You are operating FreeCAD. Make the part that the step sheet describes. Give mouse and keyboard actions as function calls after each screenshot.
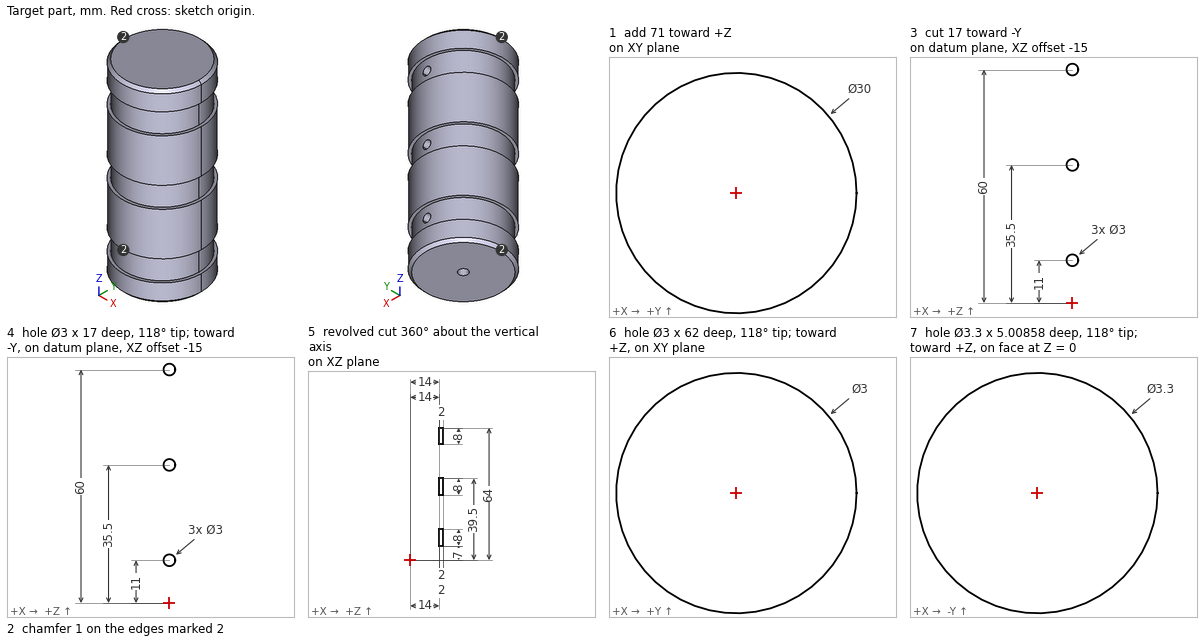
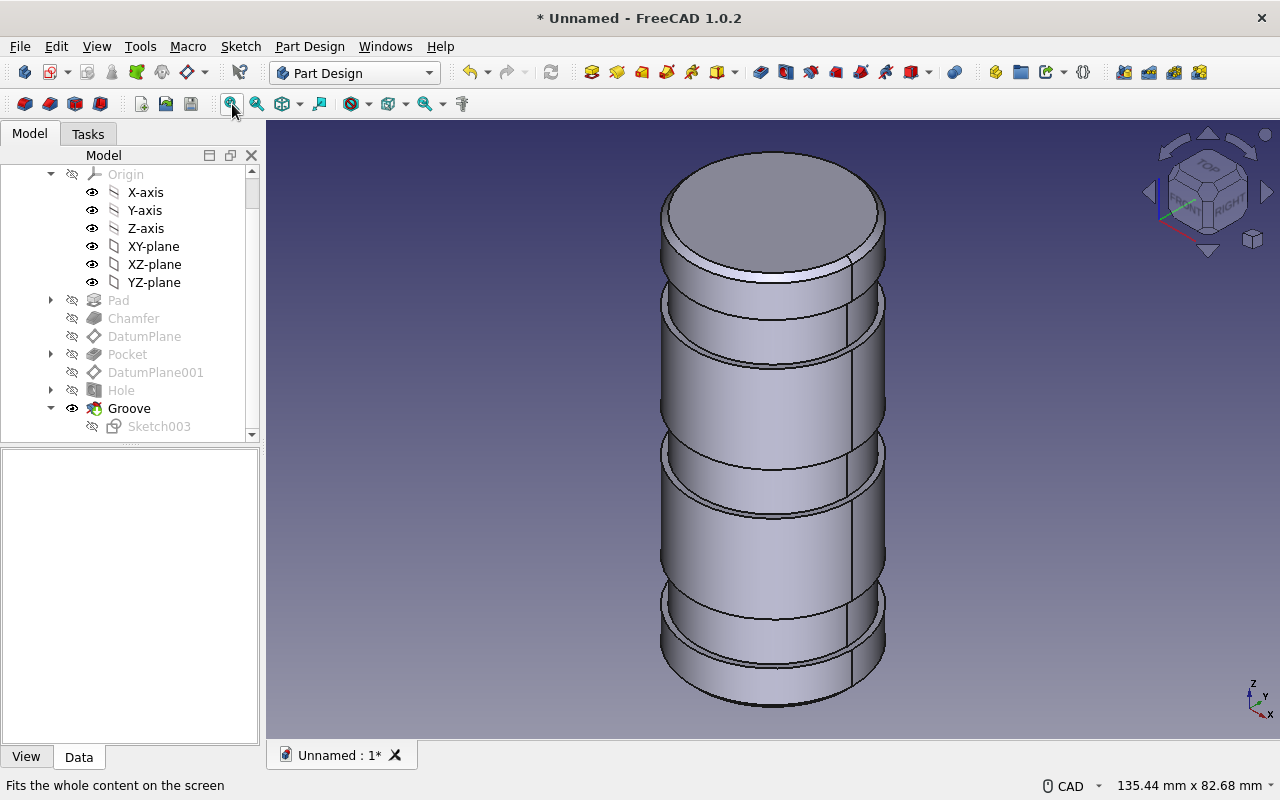
click(50, 72)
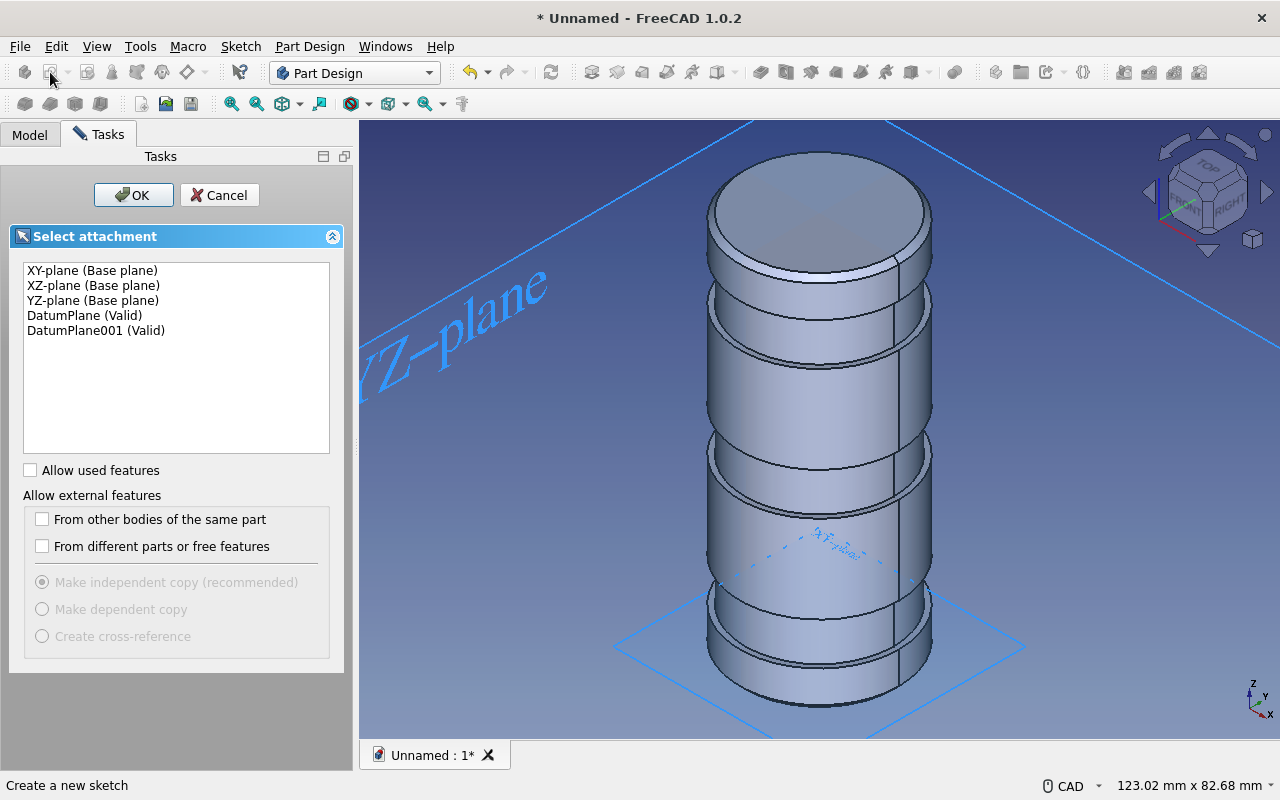
click(84, 270)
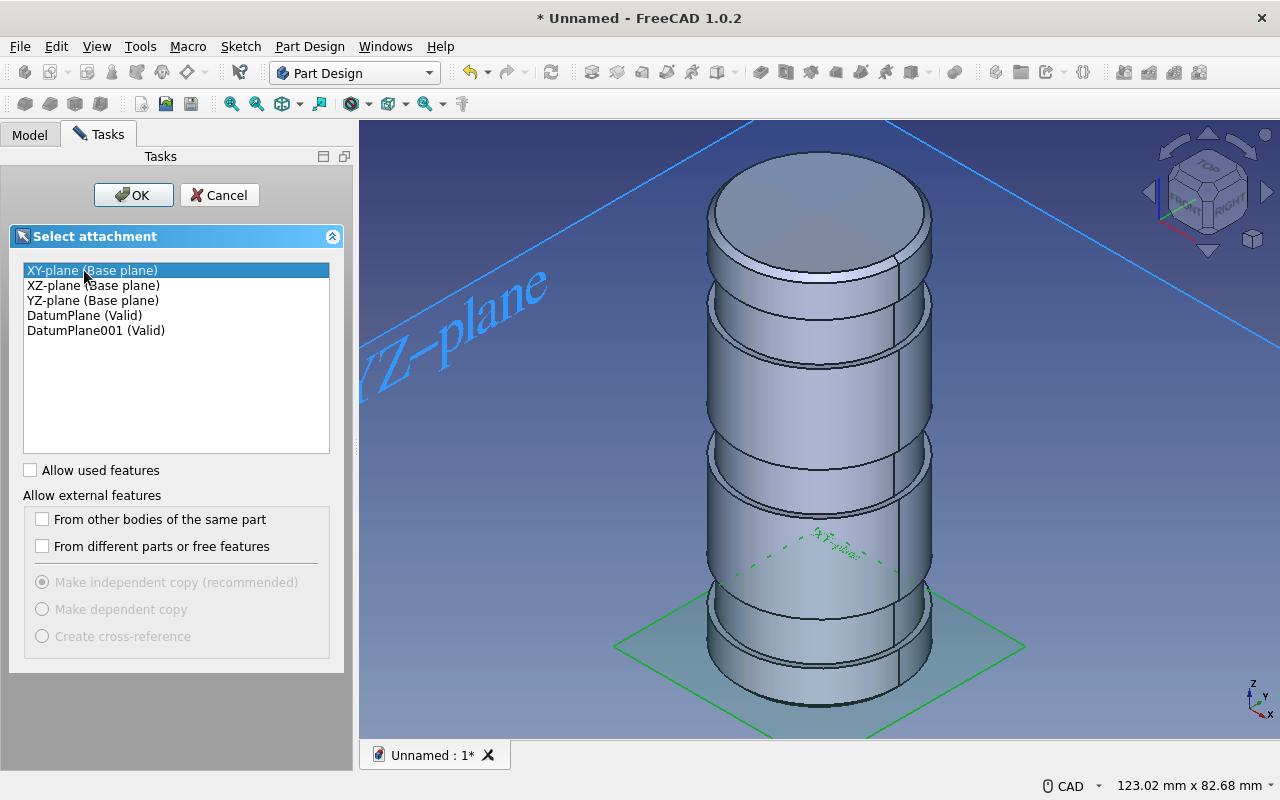
click(134, 195)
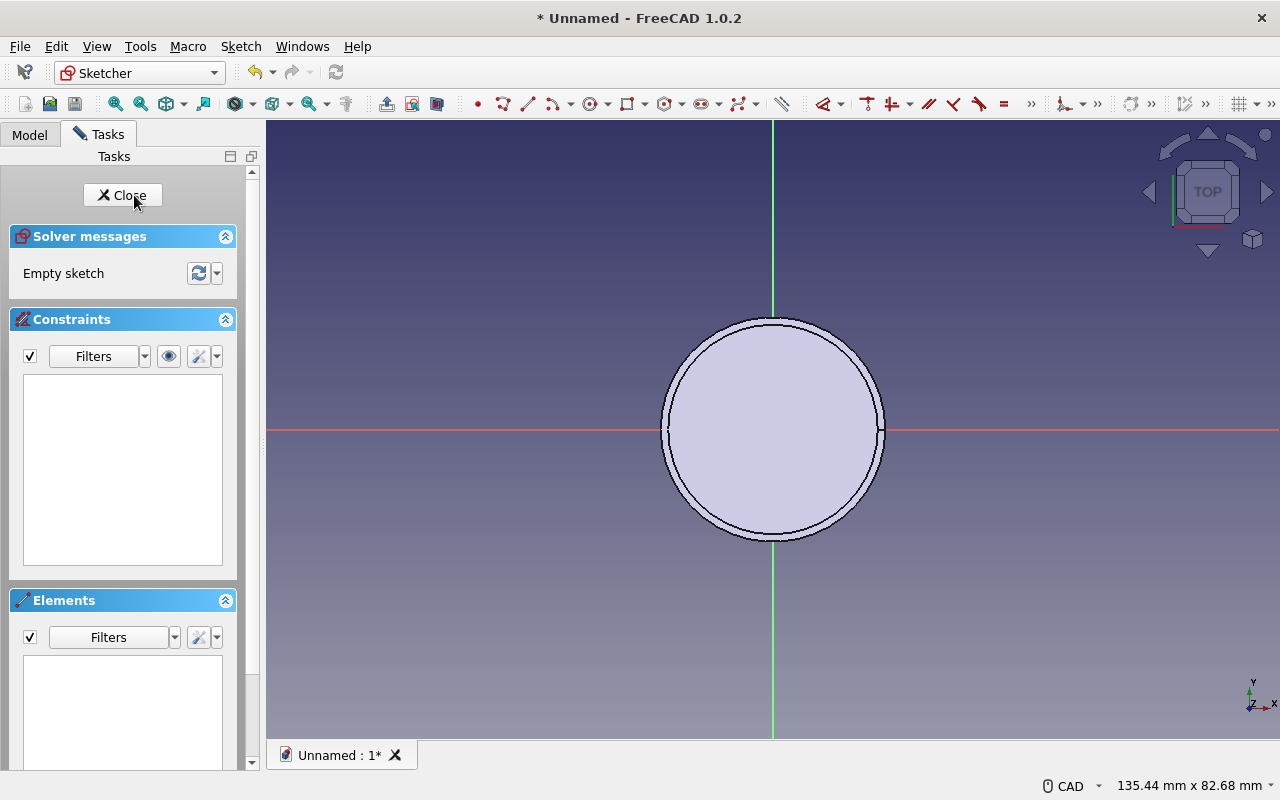
click(437, 104)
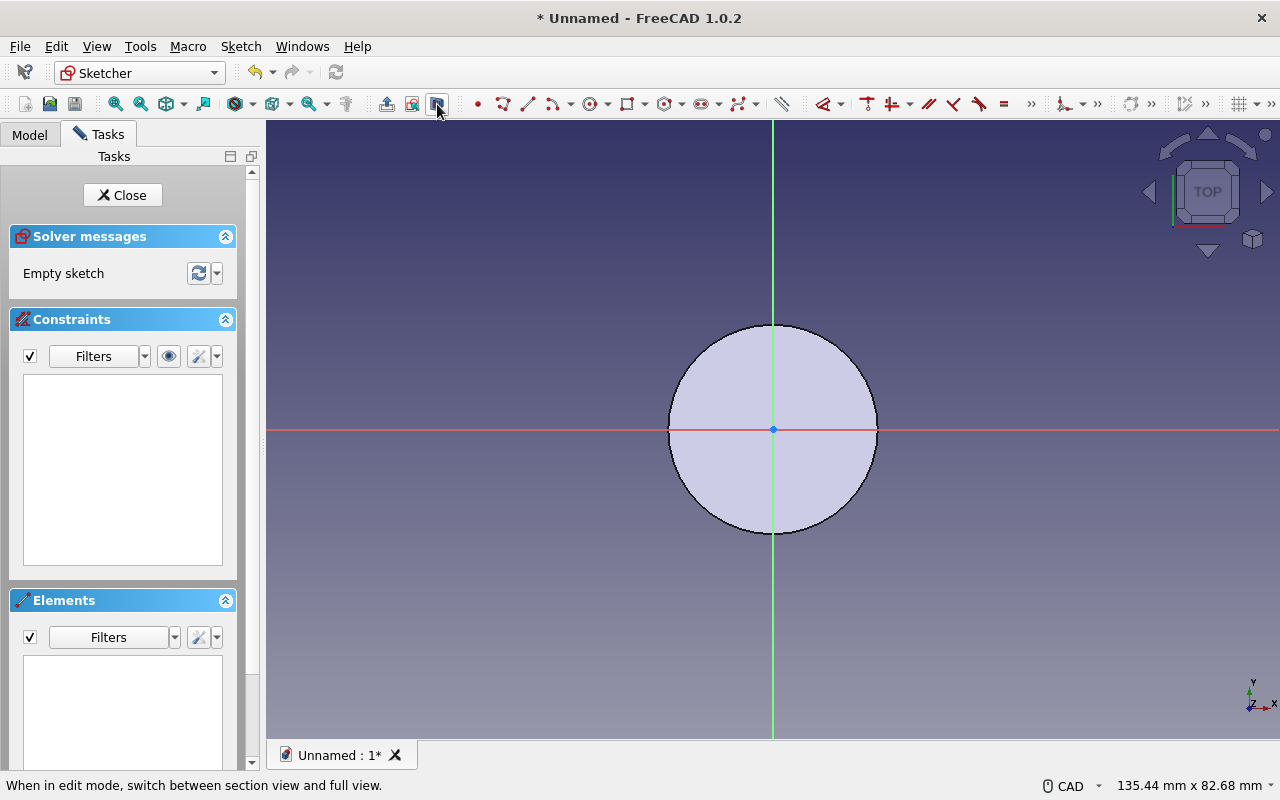
scroll(777, 430, up, 14)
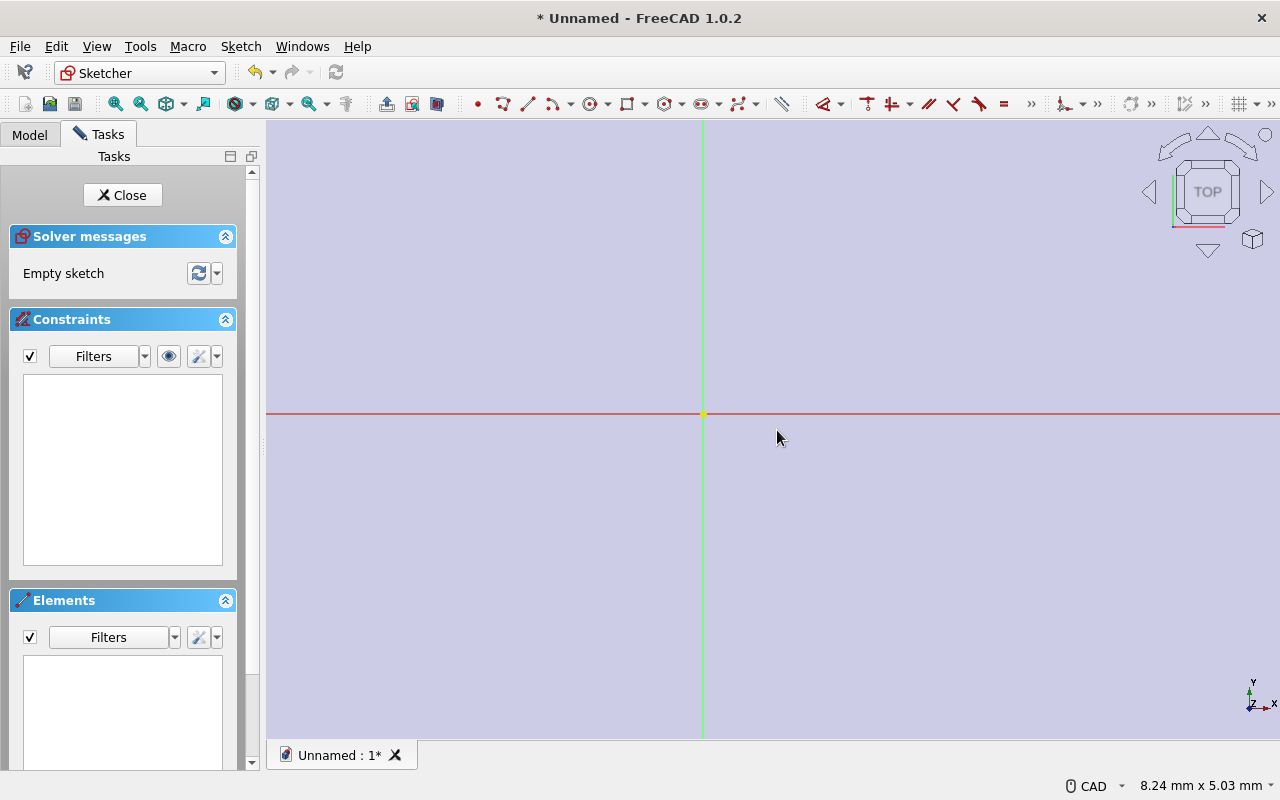
click(590, 104)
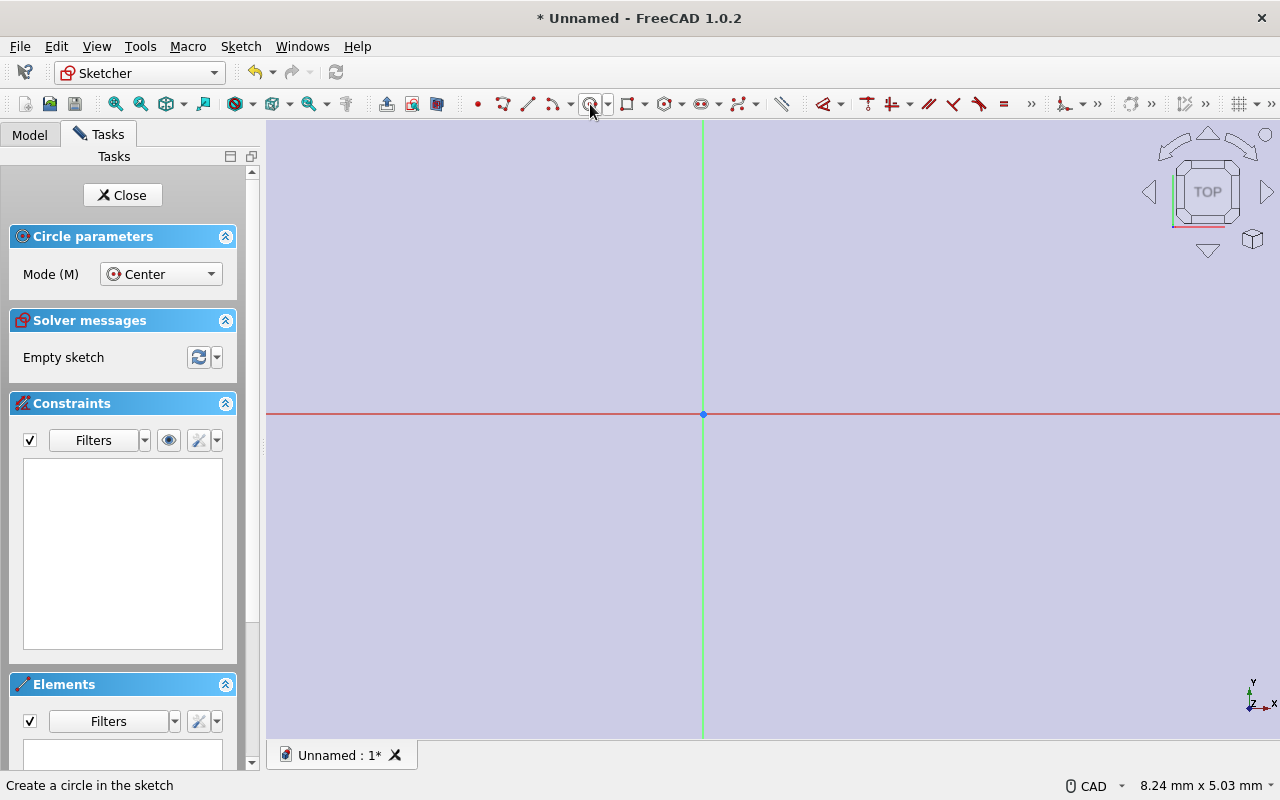
click(703, 414)
move(834, 283)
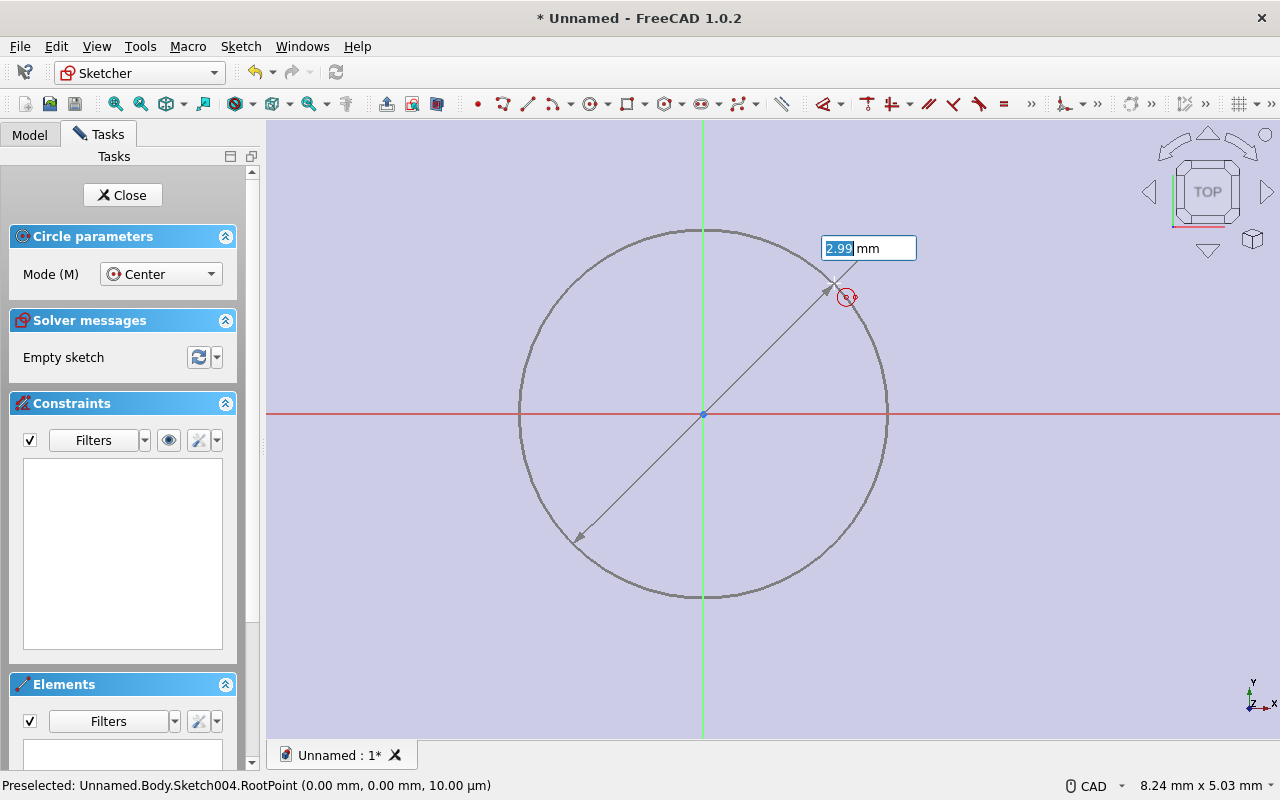
text(3)
key(Return)
key(Escape)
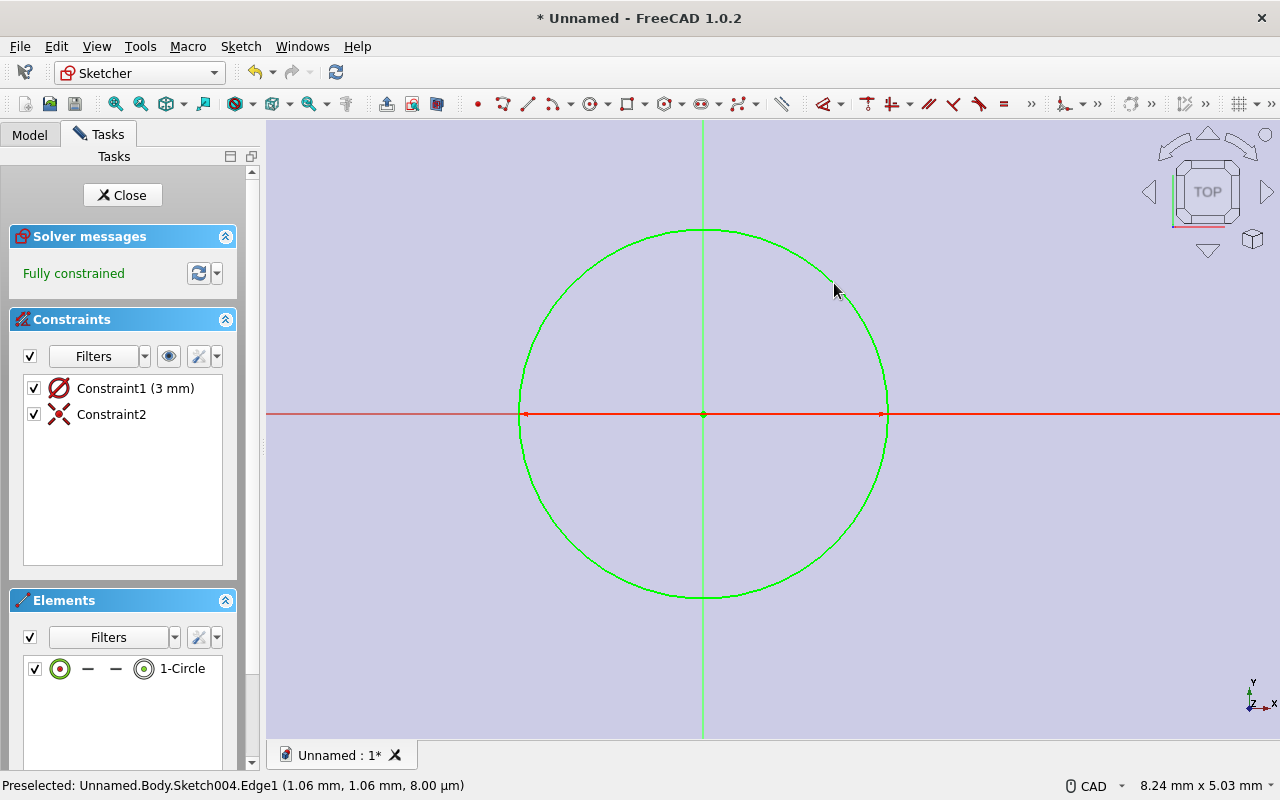
click(123, 195)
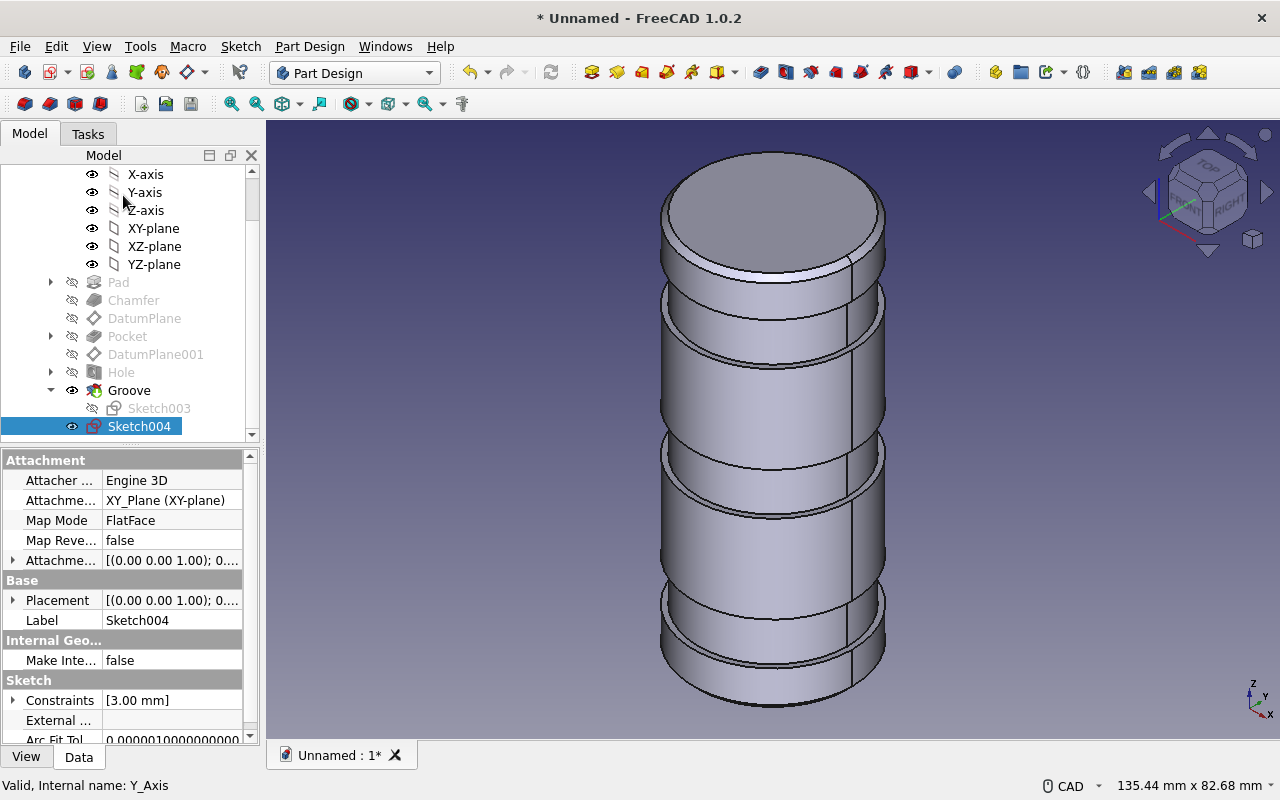
click(786, 72)